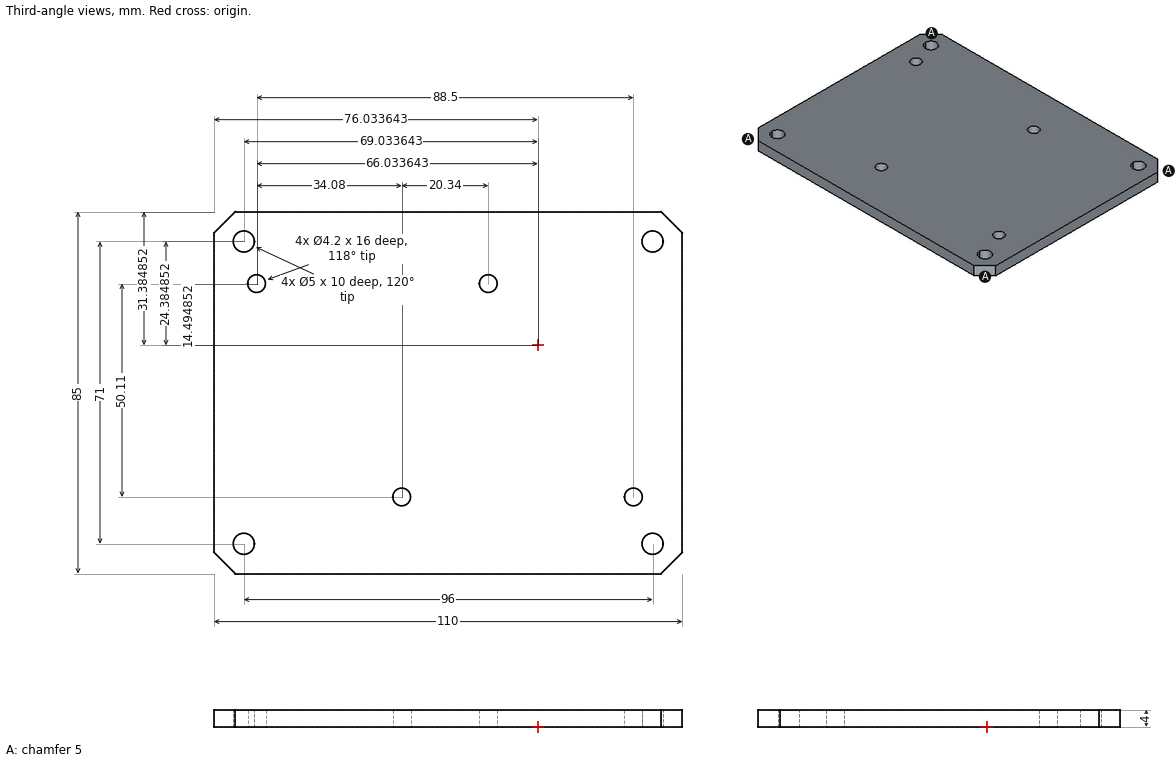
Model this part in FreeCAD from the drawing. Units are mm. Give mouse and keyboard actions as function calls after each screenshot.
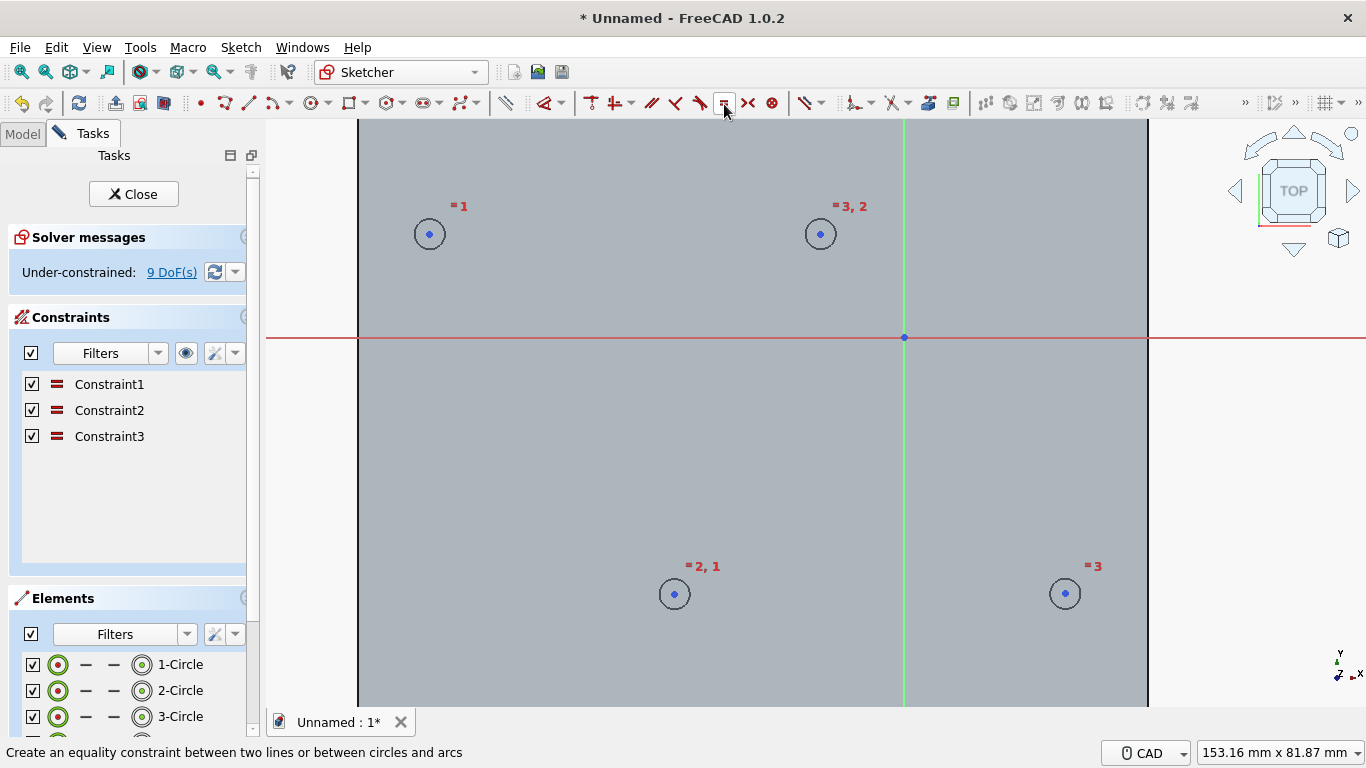
click(430, 234)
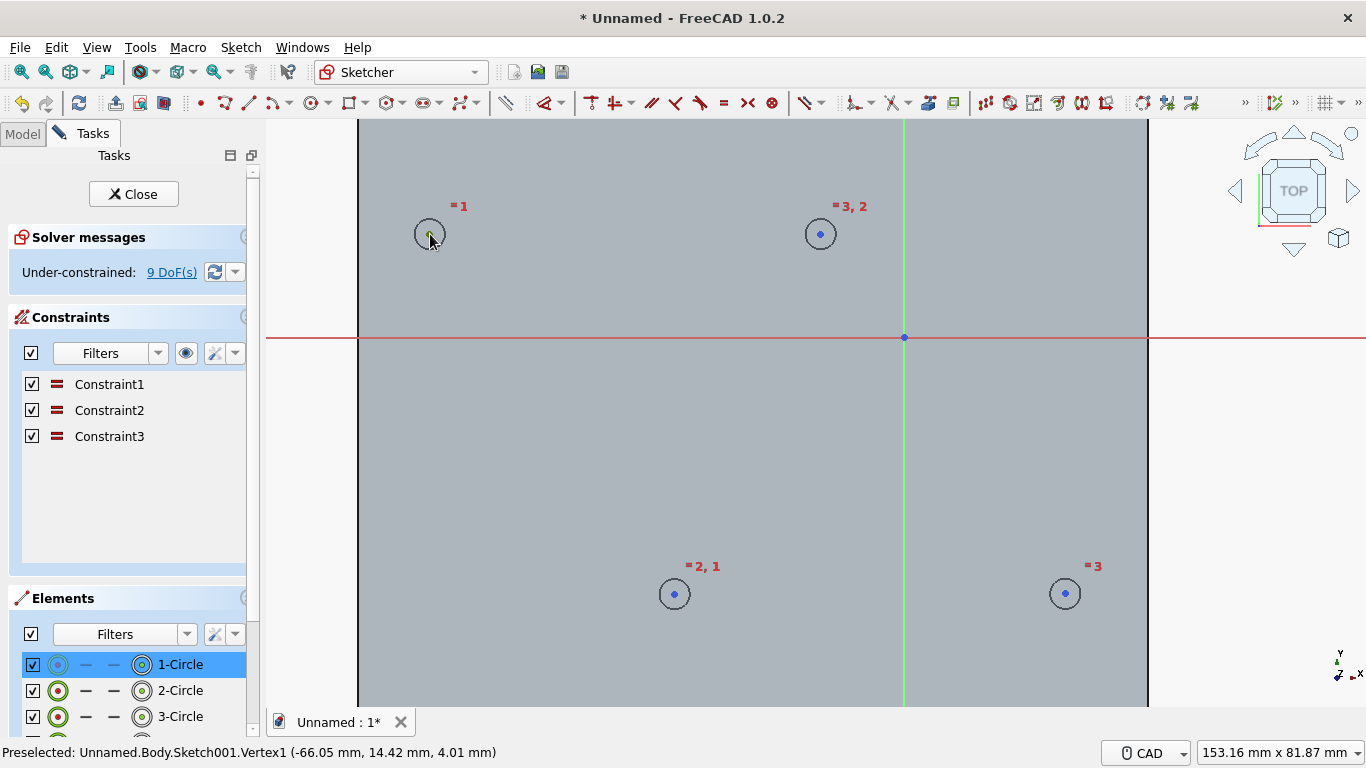
click(821, 234)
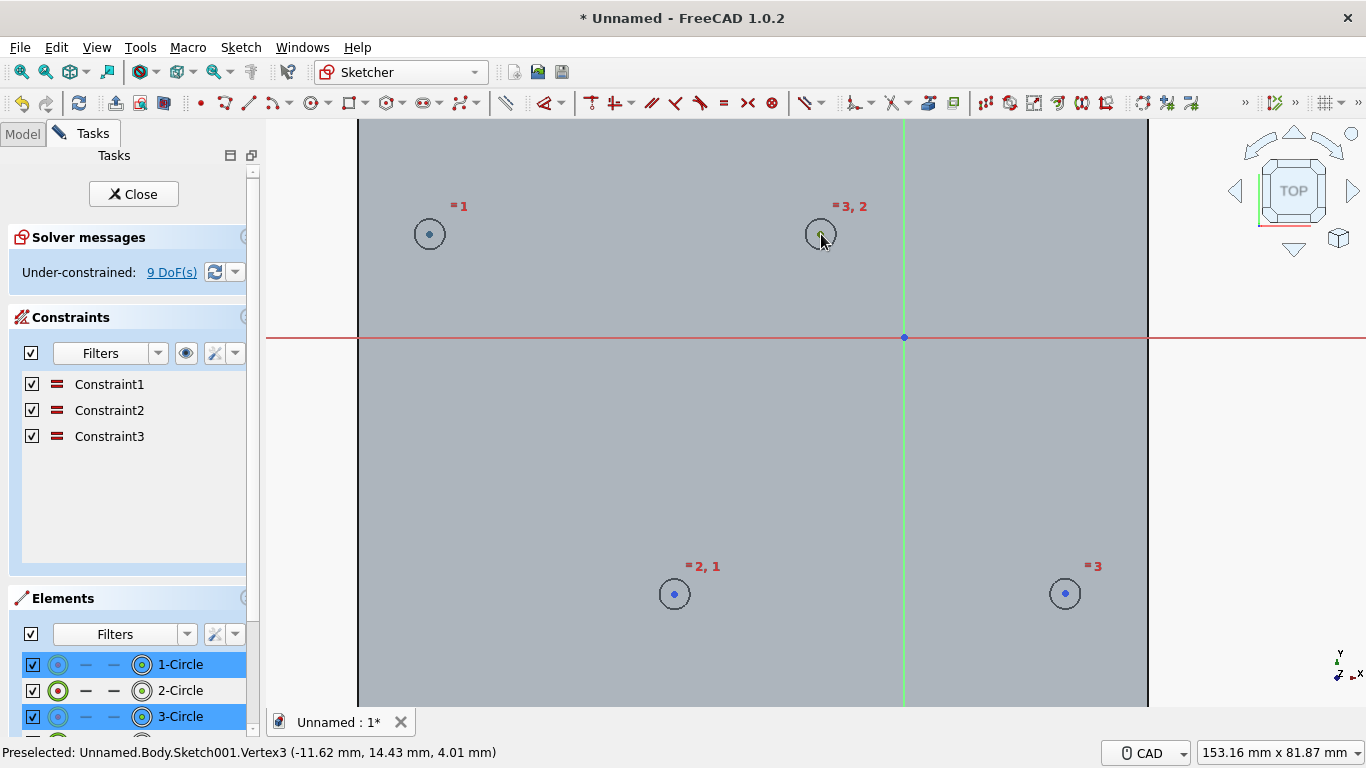
key(h)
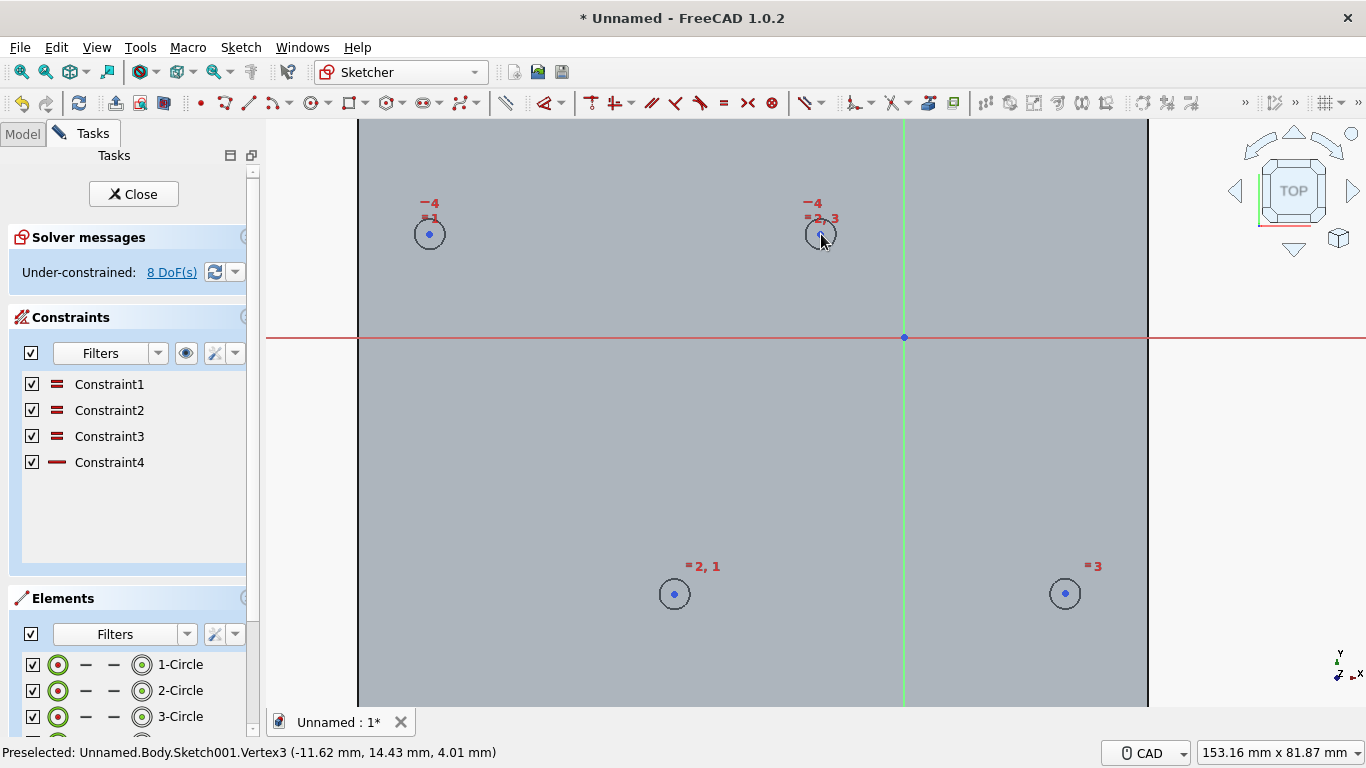
click(675, 594)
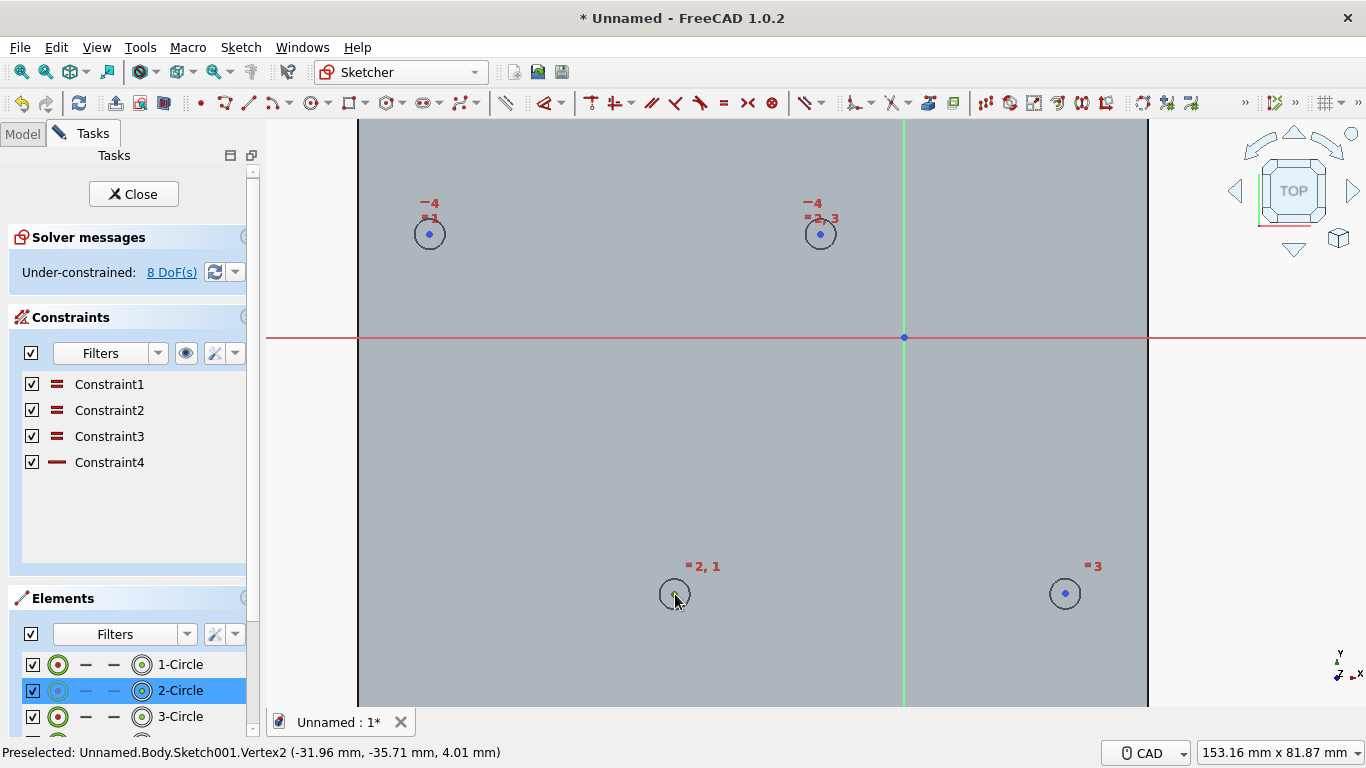
click(1065, 594)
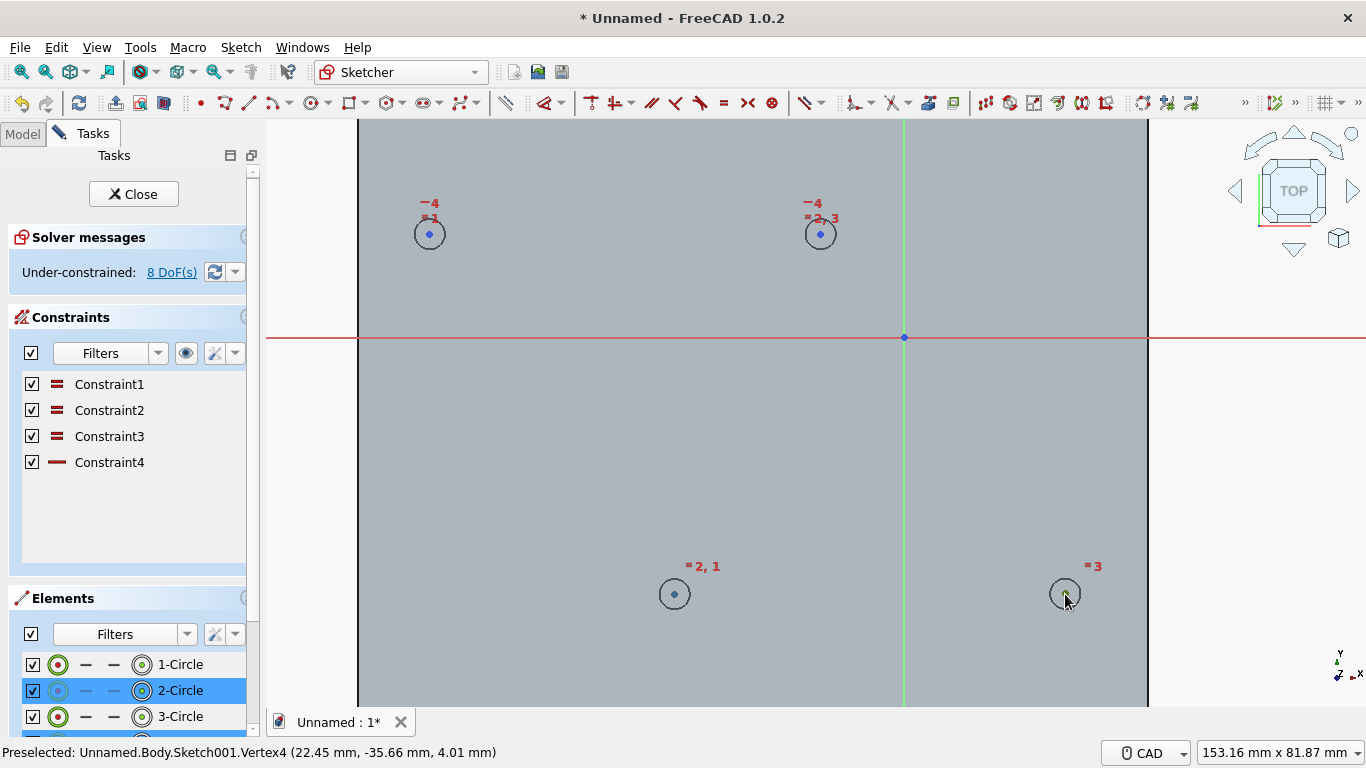
click(634, 104)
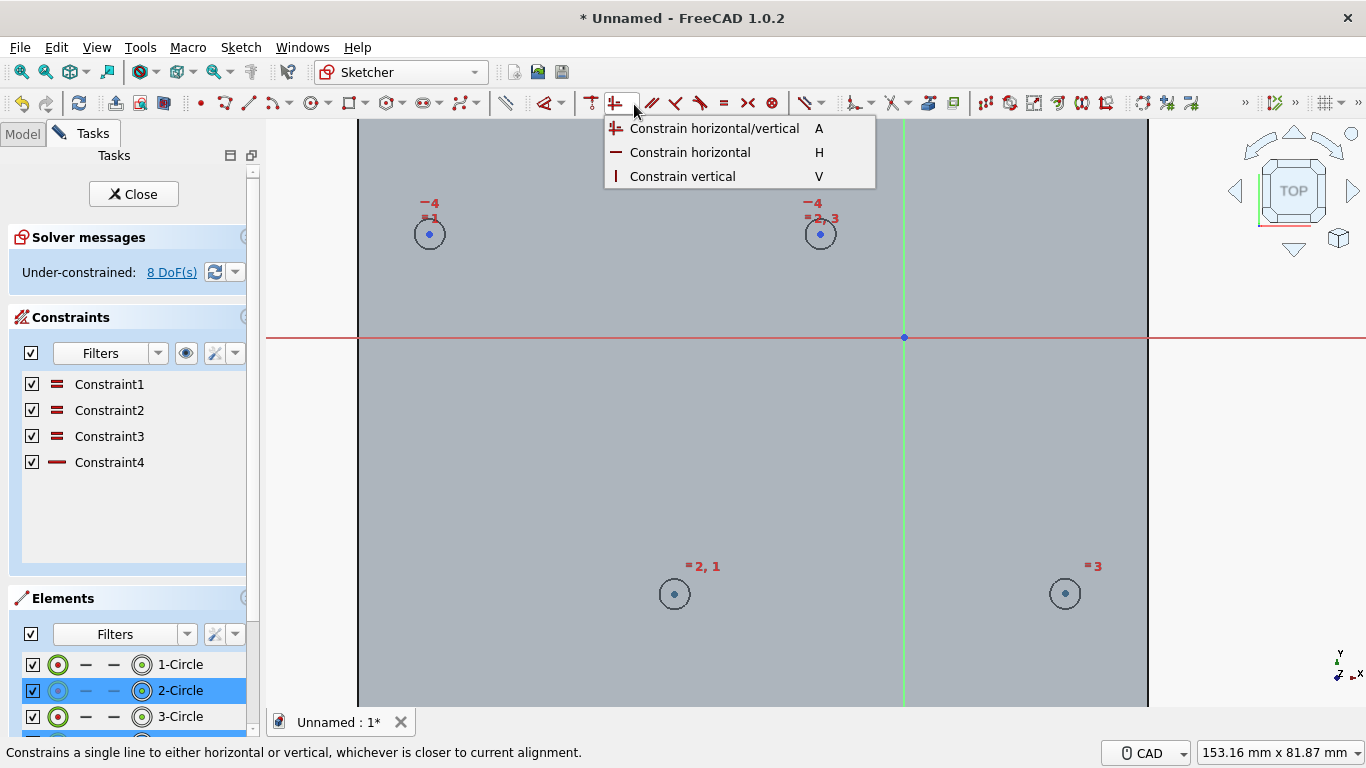
click(740, 152)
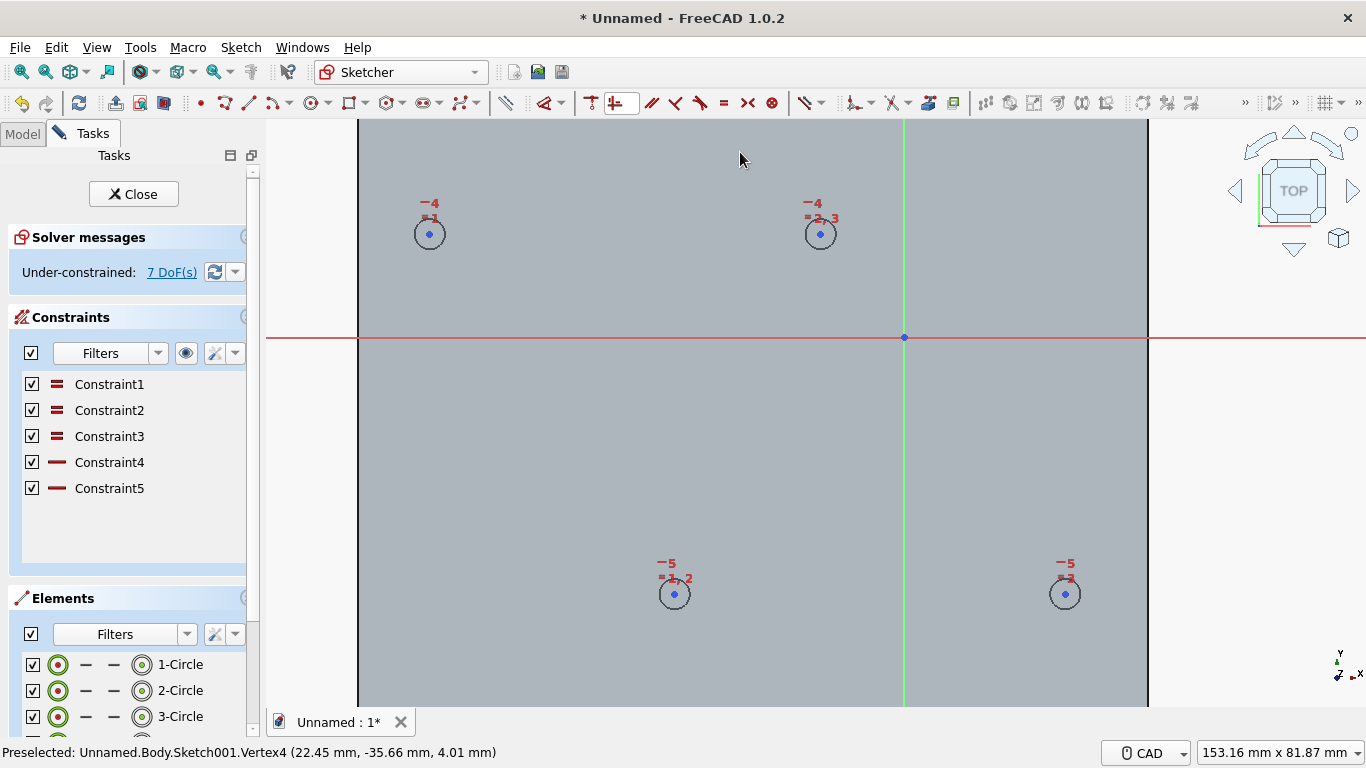
click(544, 104)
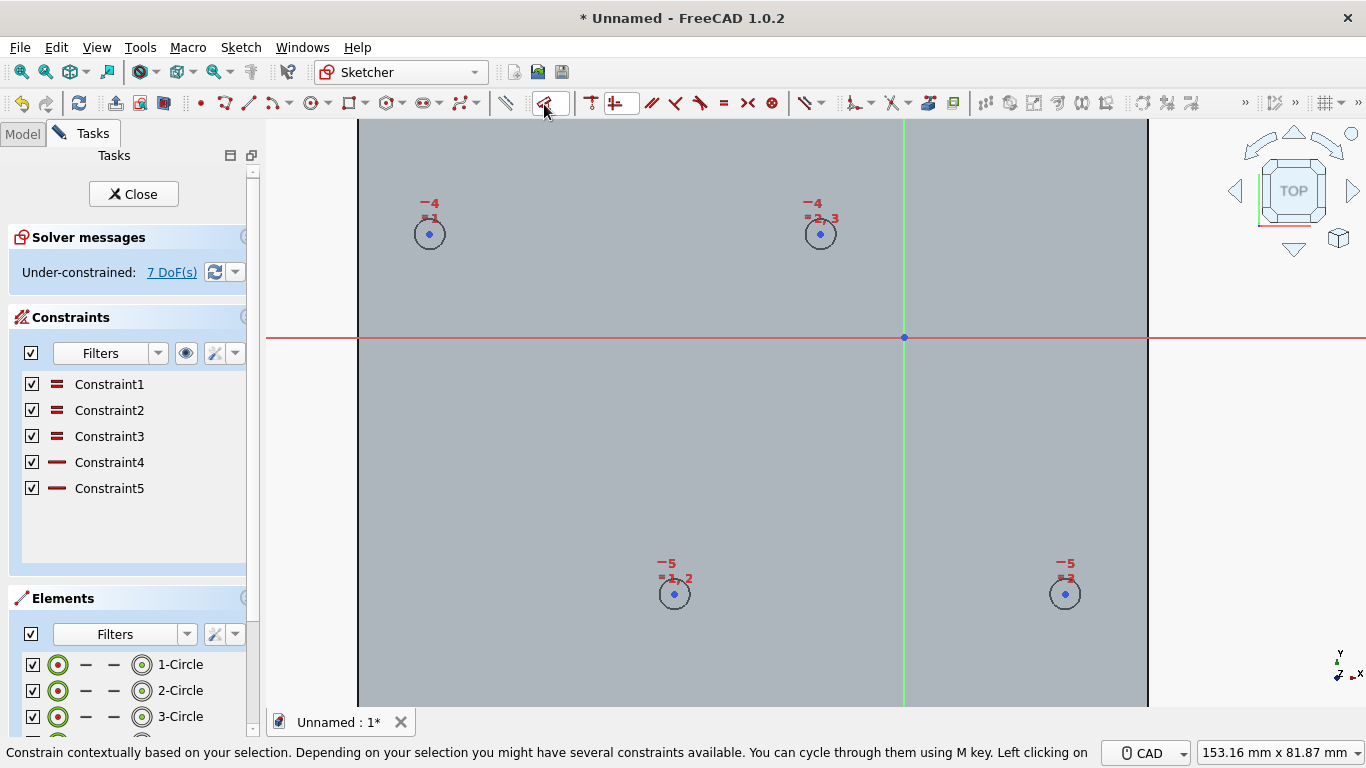
scroll(440, 223, up, 2)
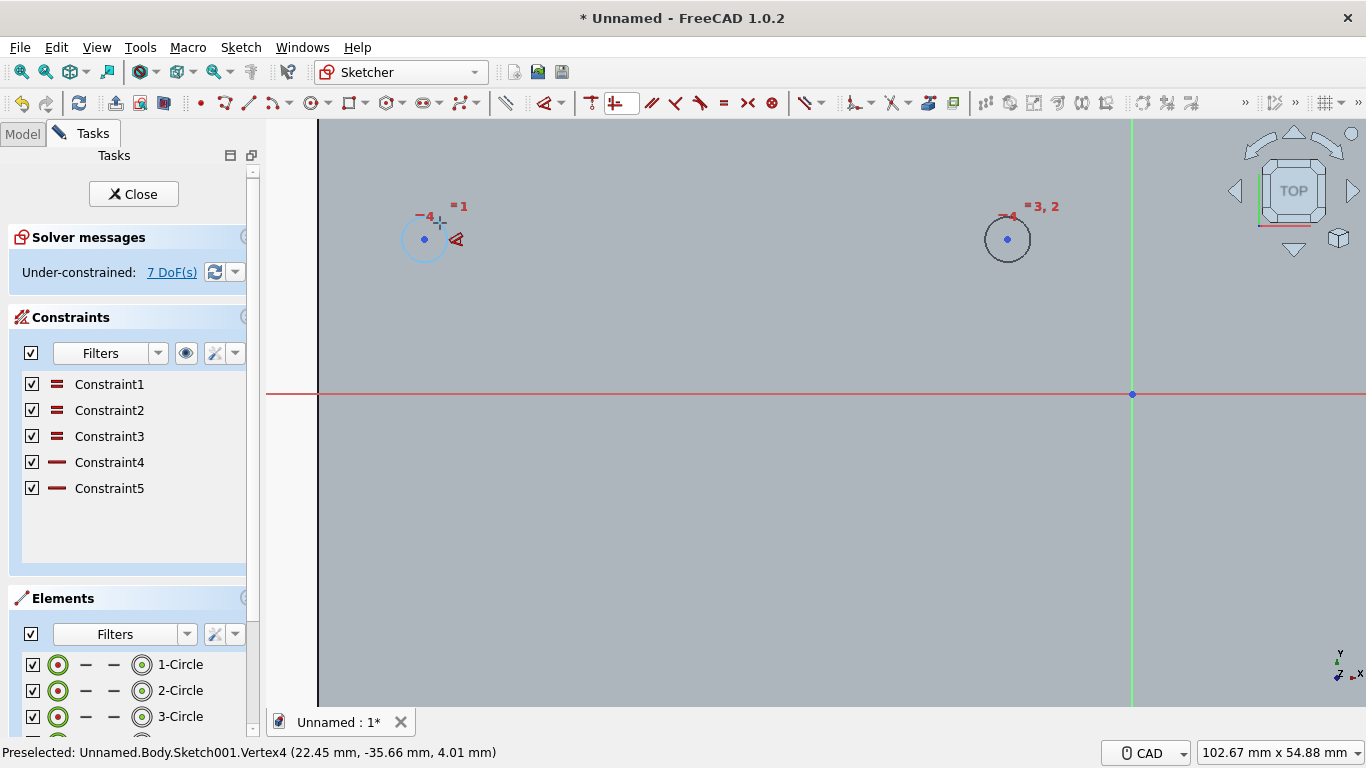
click(441, 224)
click(464, 202)